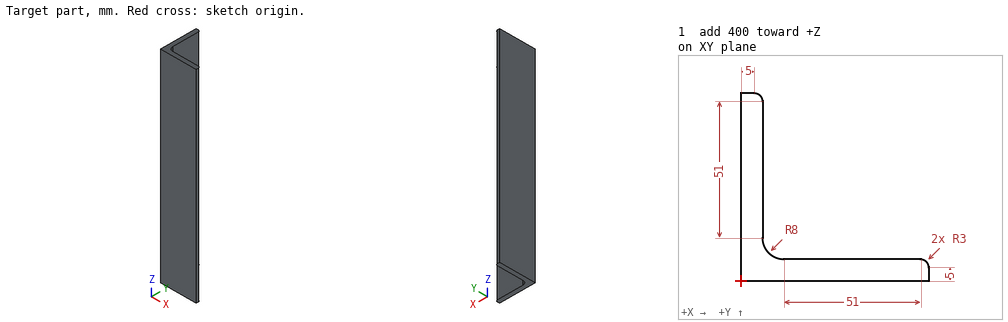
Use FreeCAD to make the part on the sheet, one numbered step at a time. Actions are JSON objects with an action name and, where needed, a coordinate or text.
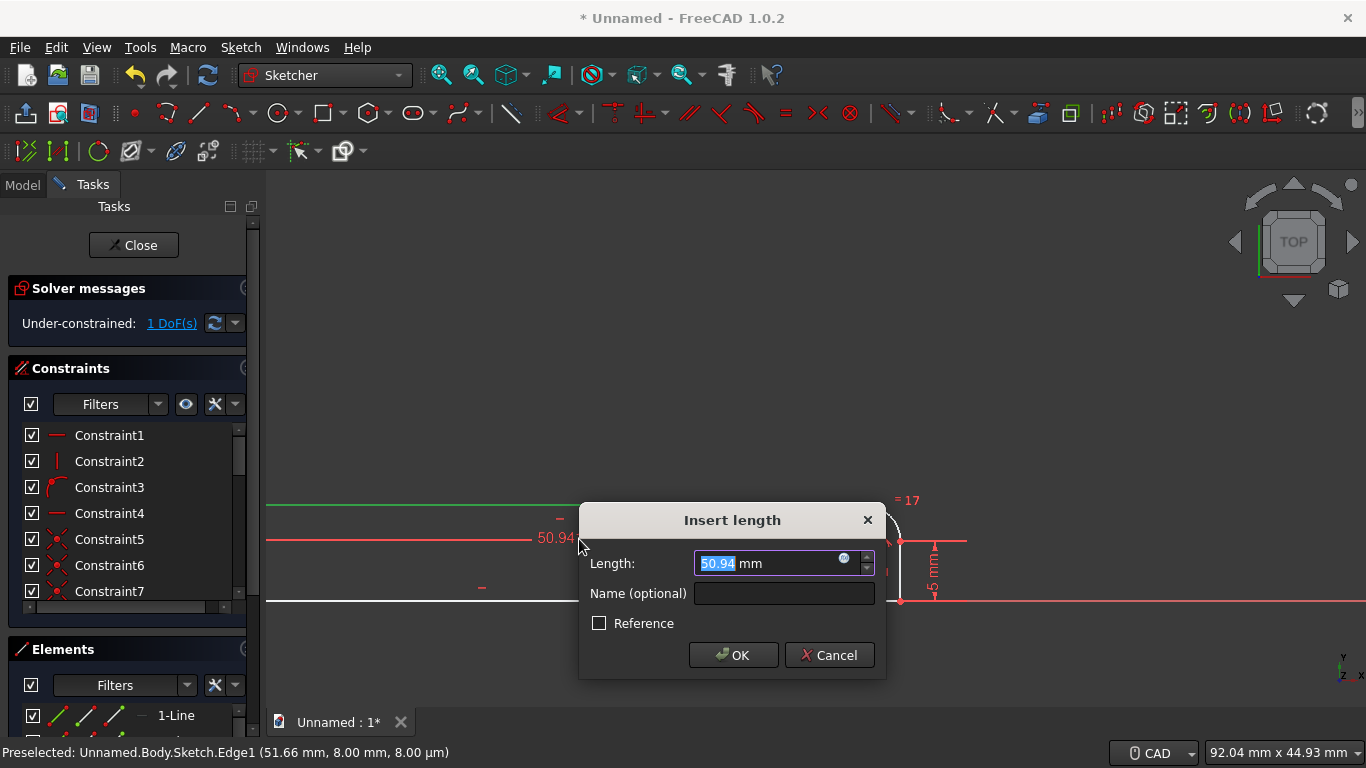
{"action": "type", "text": "51"}
{"action": "key", "text": "Return"}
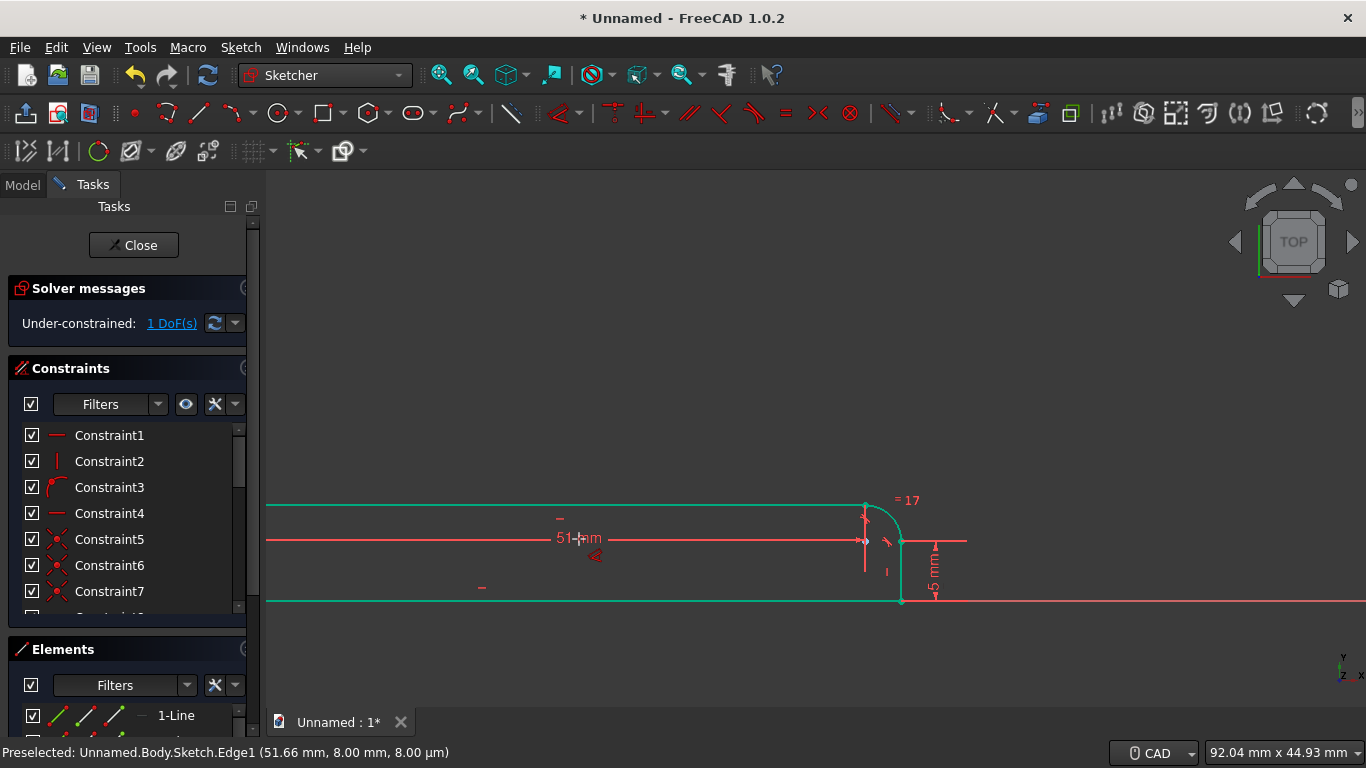
{"action": "scroll", "coordinate": [901, 587], "scroll_direction": "down", "scroll_amount": 5}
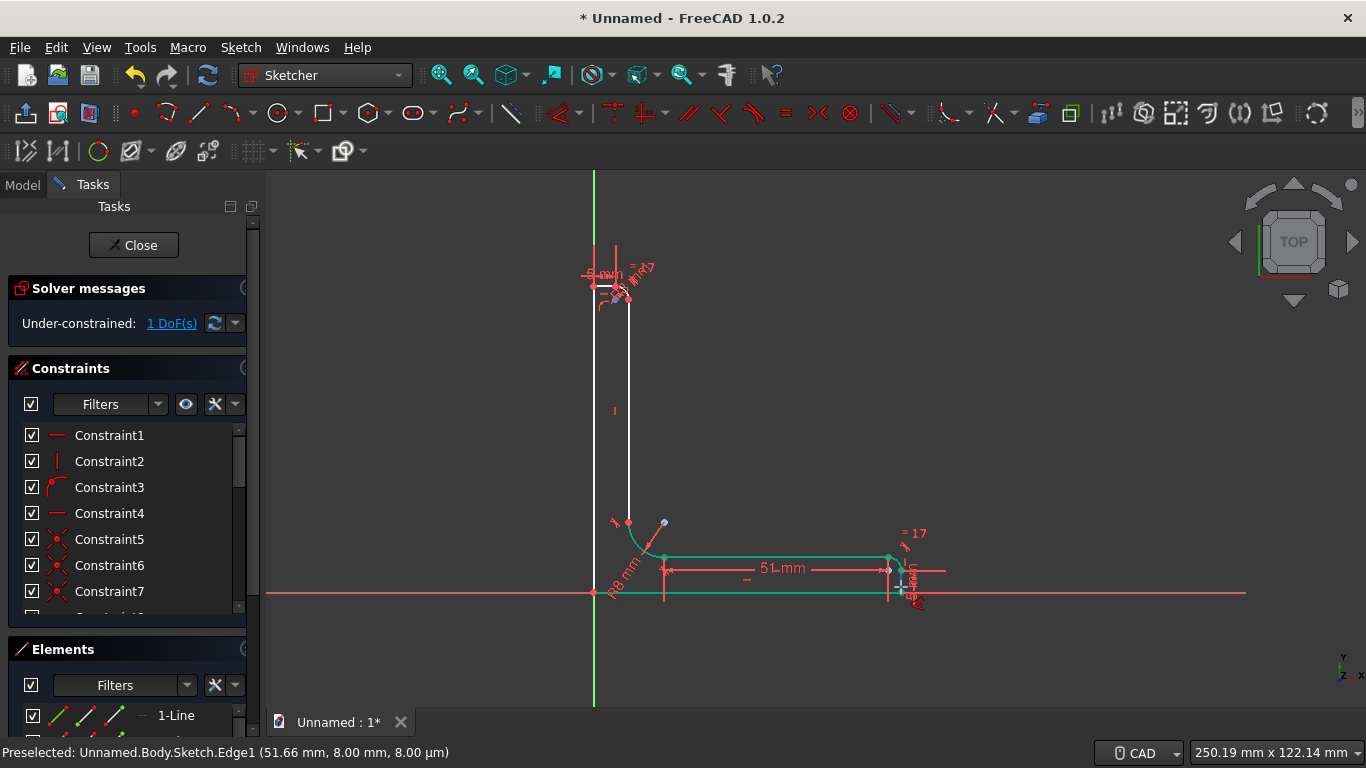
{"action": "left_click", "coordinate": [629, 455]}
{"action": "left_click", "coordinate": [663, 411]}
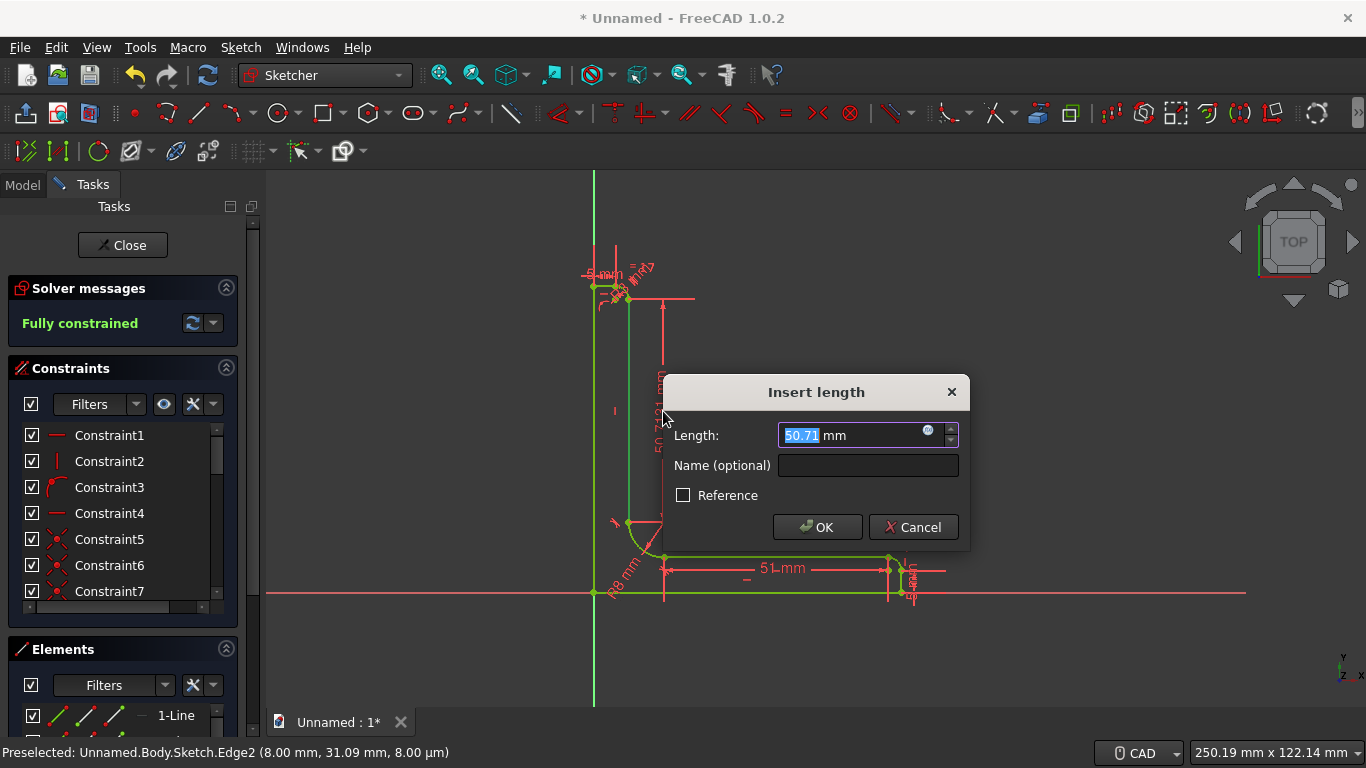
{"action": "type", "text": "51"}
{"action": "key", "text": "Return"}
{"action": "key", "text": "Escape"}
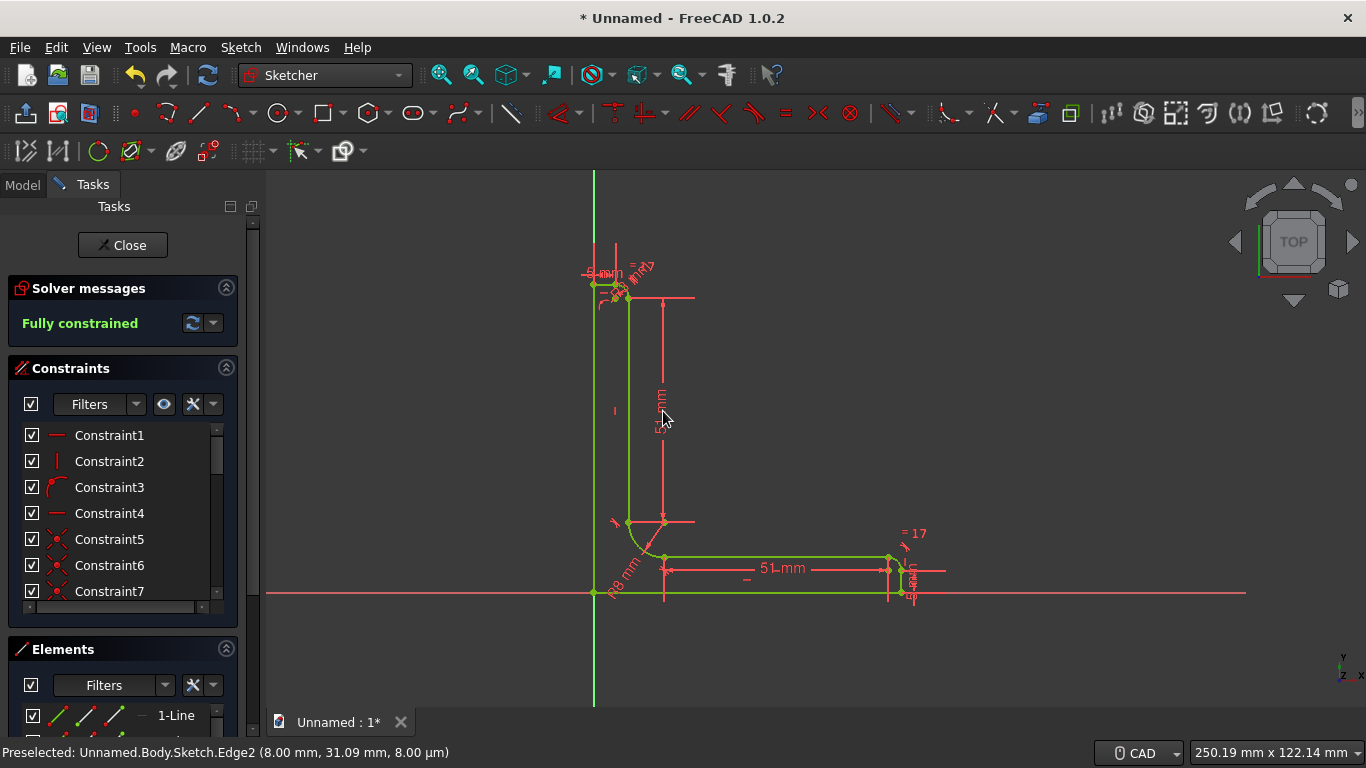
{"action": "left_click", "coordinate": [123, 245]}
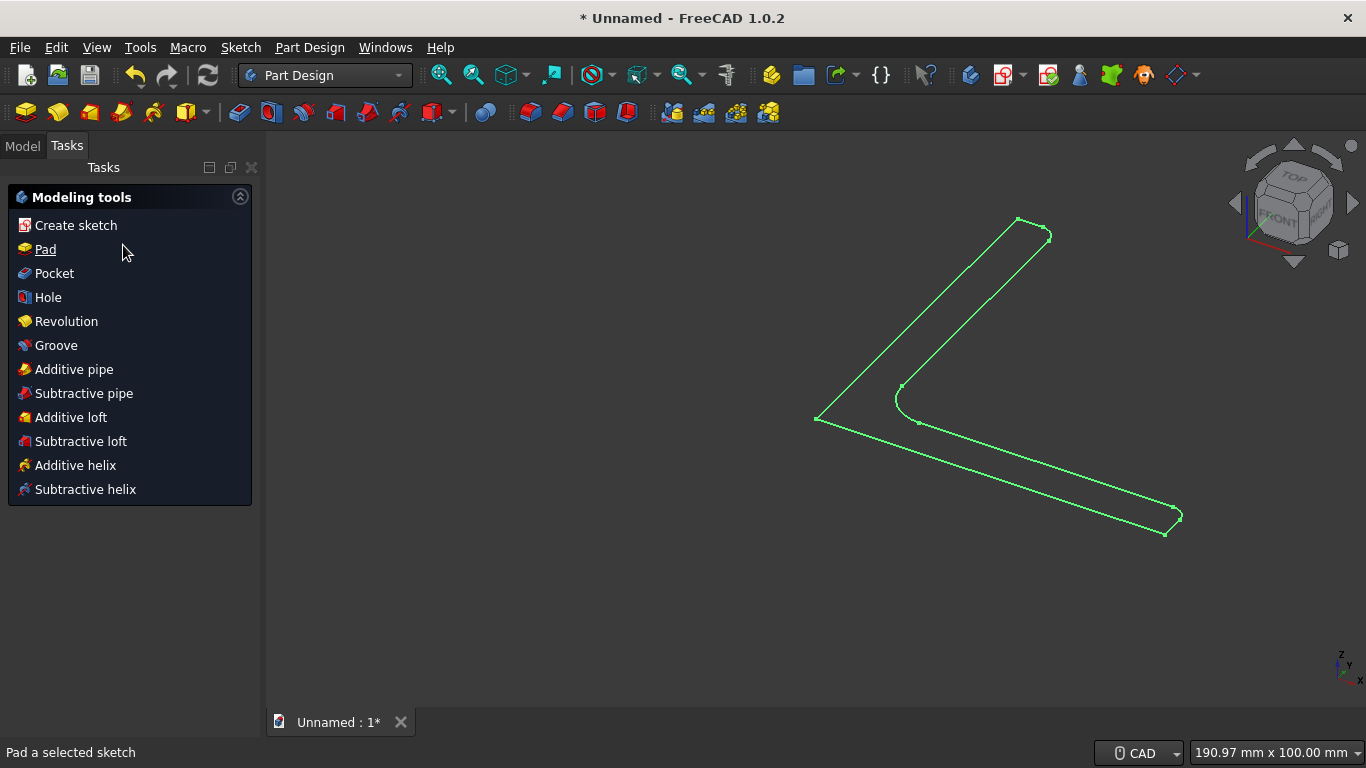
{"action": "left_click", "coordinate": [26, 112]}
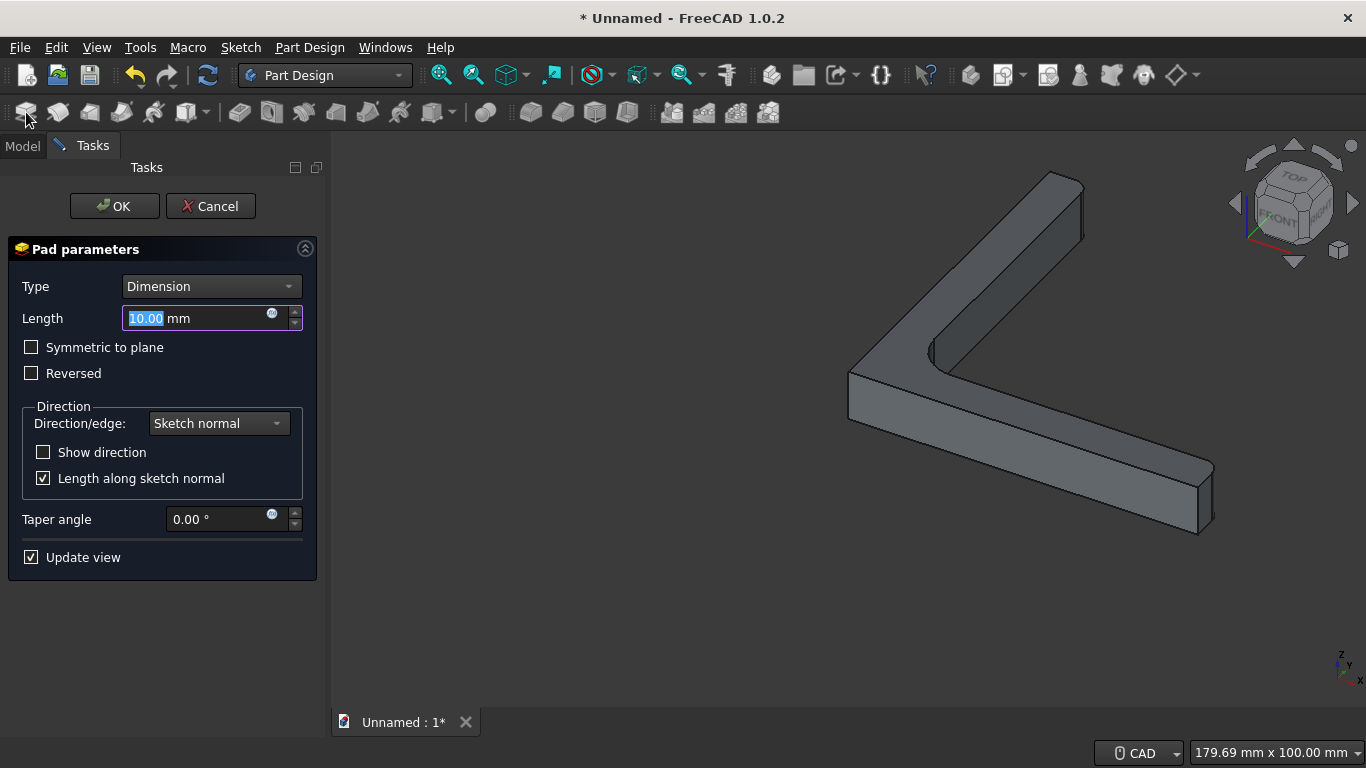
{"action": "type", "text": "400"}
{"action": "key", "text": "Tab"}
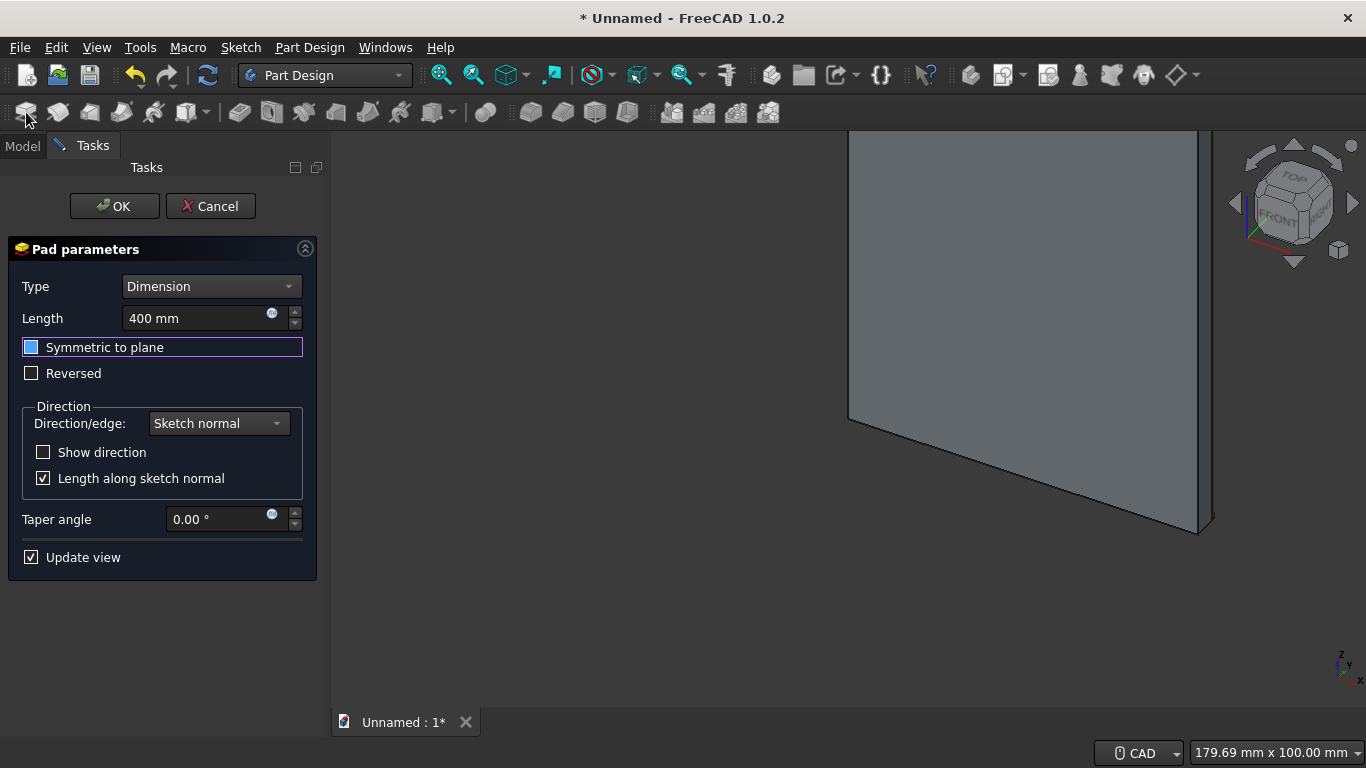
{"action": "left_click", "coordinate": [115, 206]}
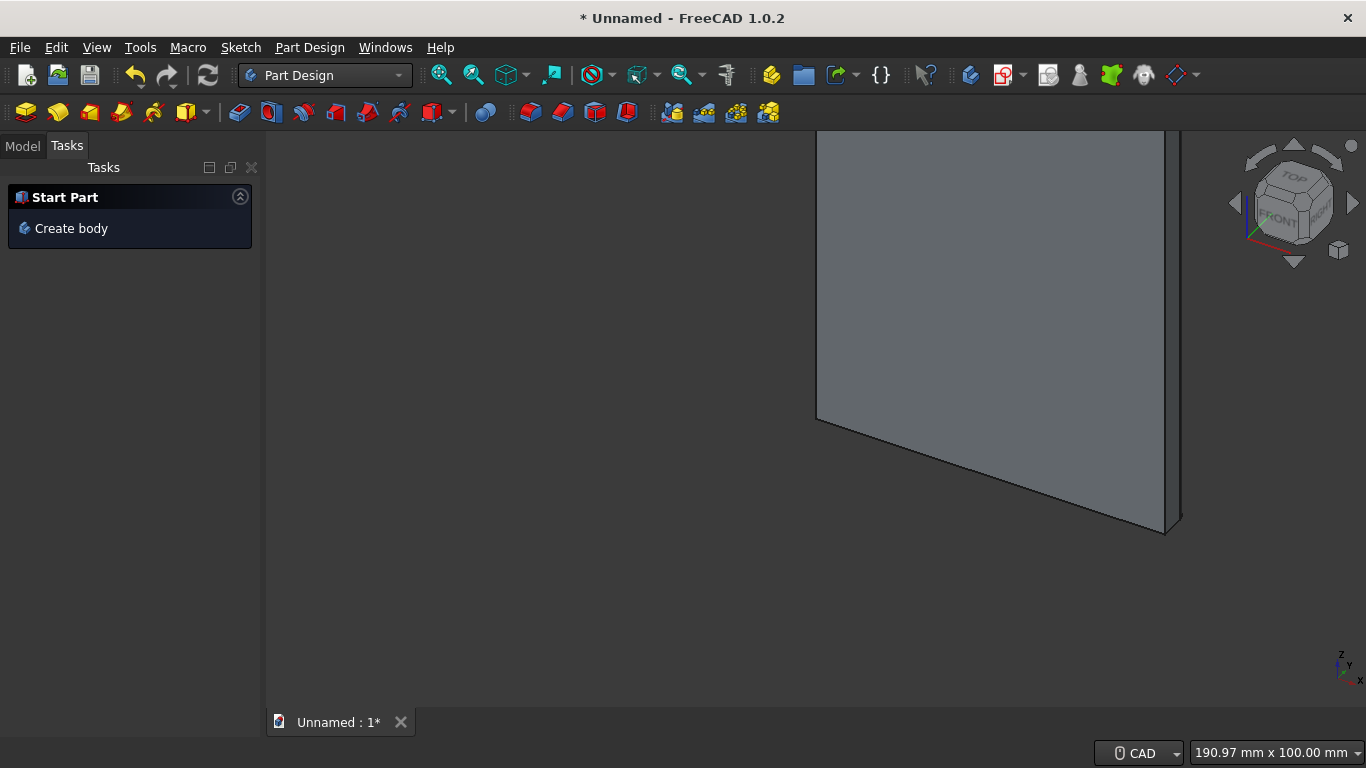
{"action": "key", "text": "0"}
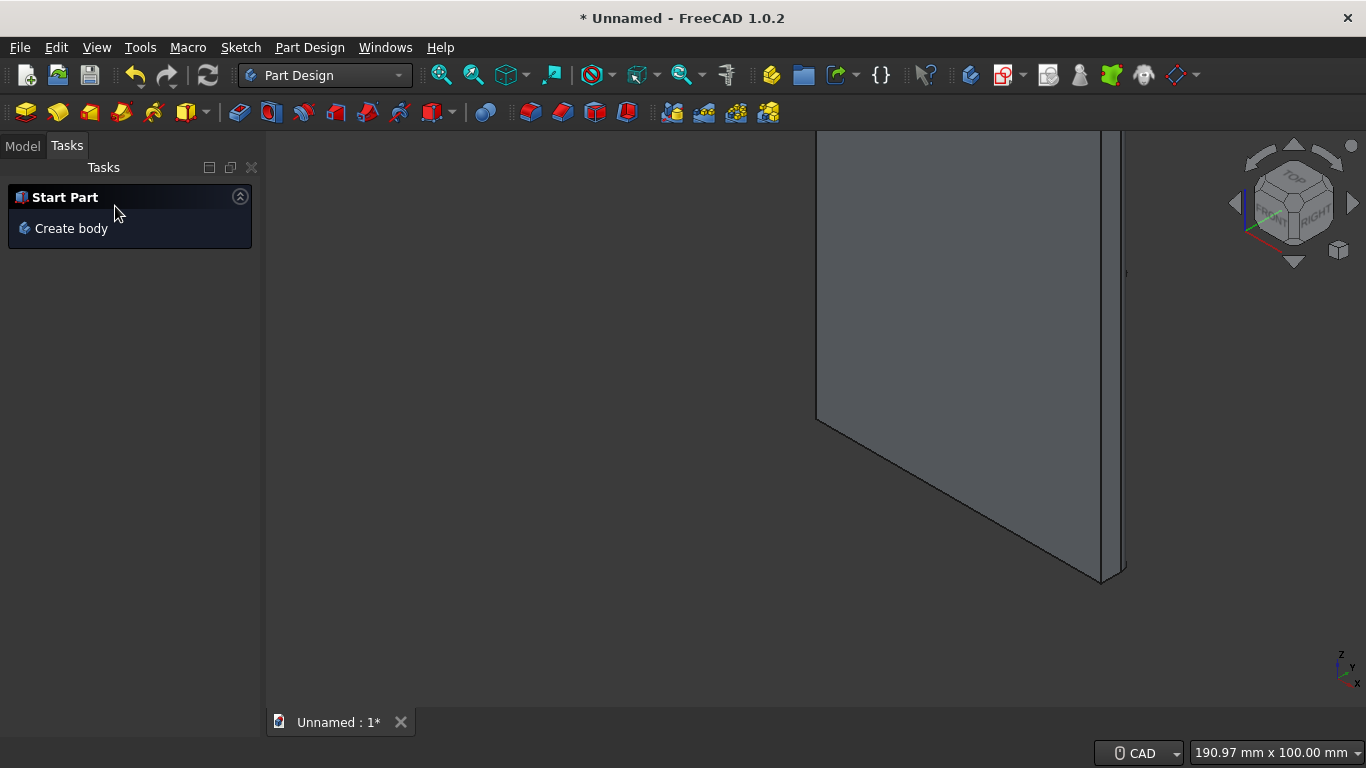
{"action": "left_click", "coordinate": [442, 76]}